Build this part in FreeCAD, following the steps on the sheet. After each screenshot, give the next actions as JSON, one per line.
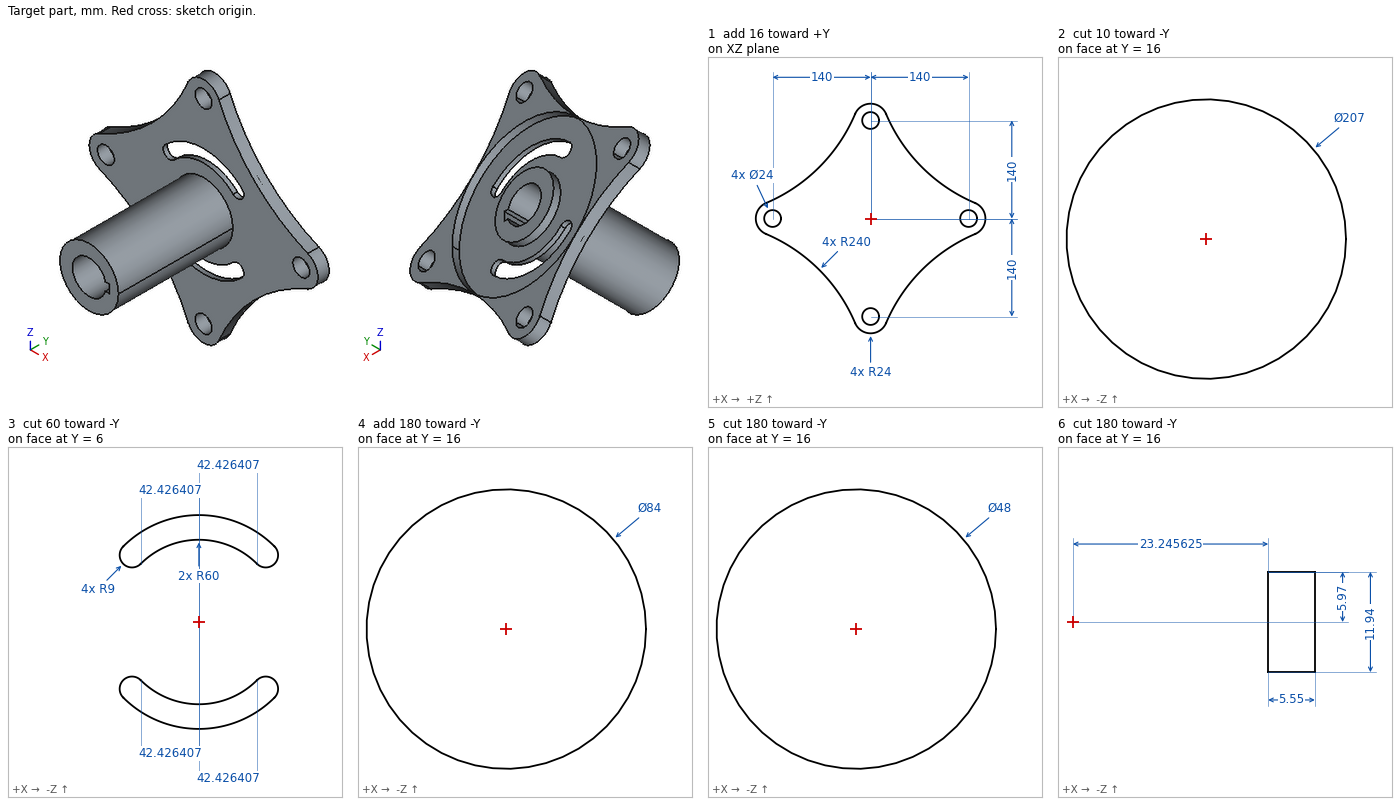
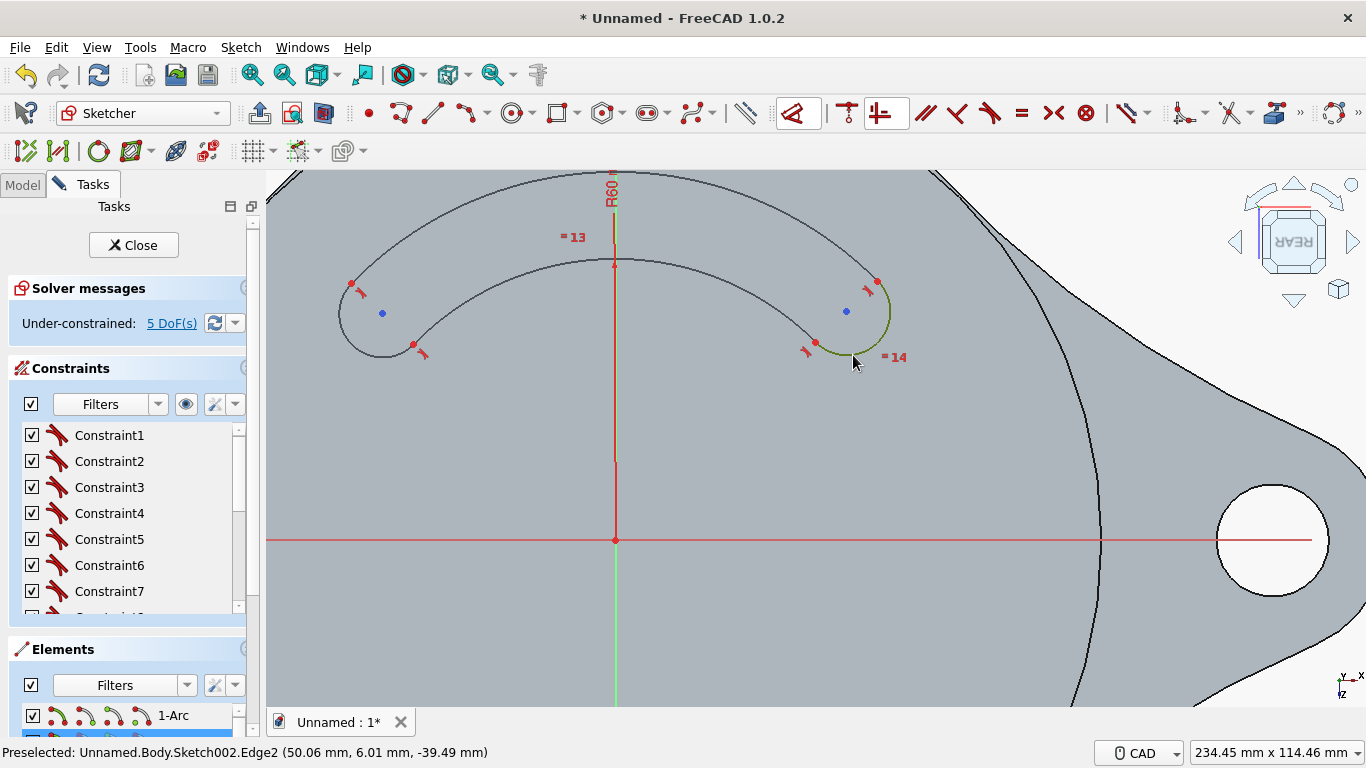
{"action": "key", "text": "k r"}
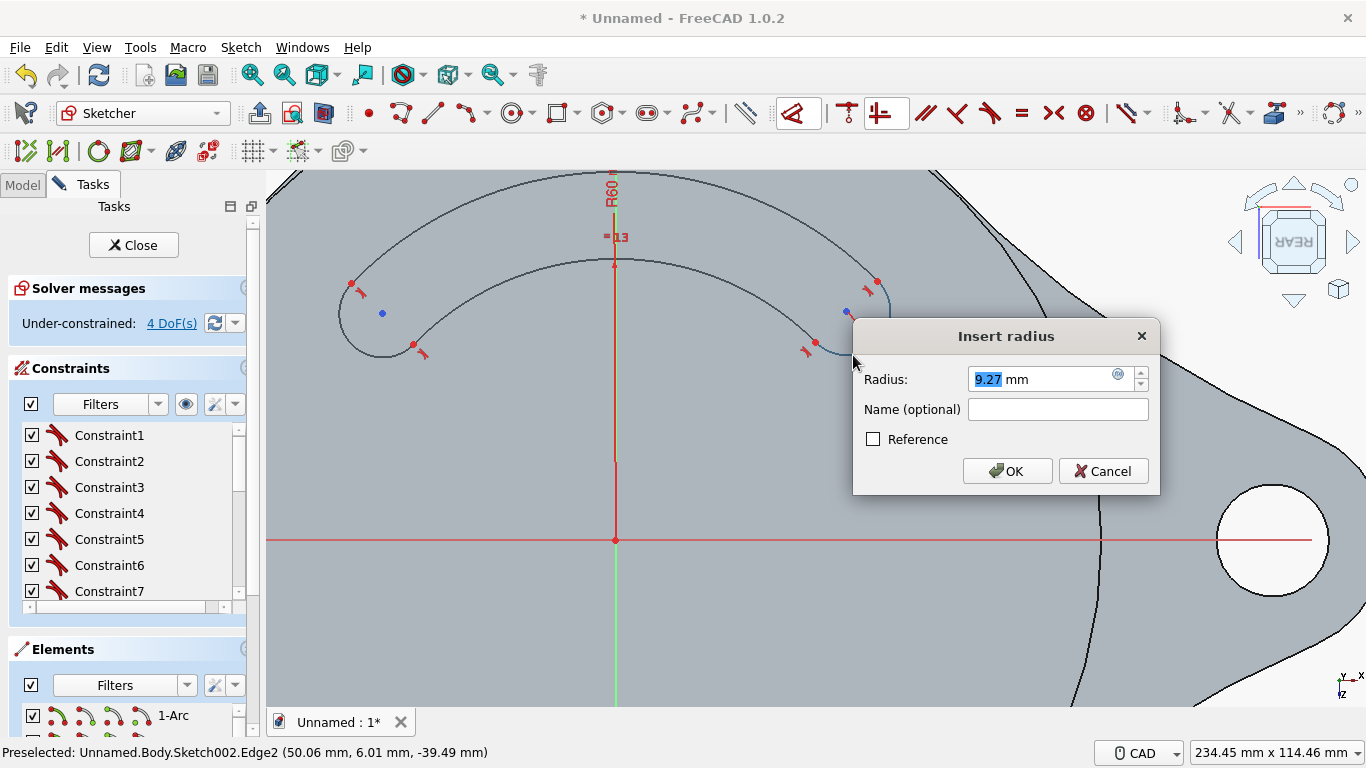
{"action": "type", "text": "9"}
{"action": "key", "text": "Return"}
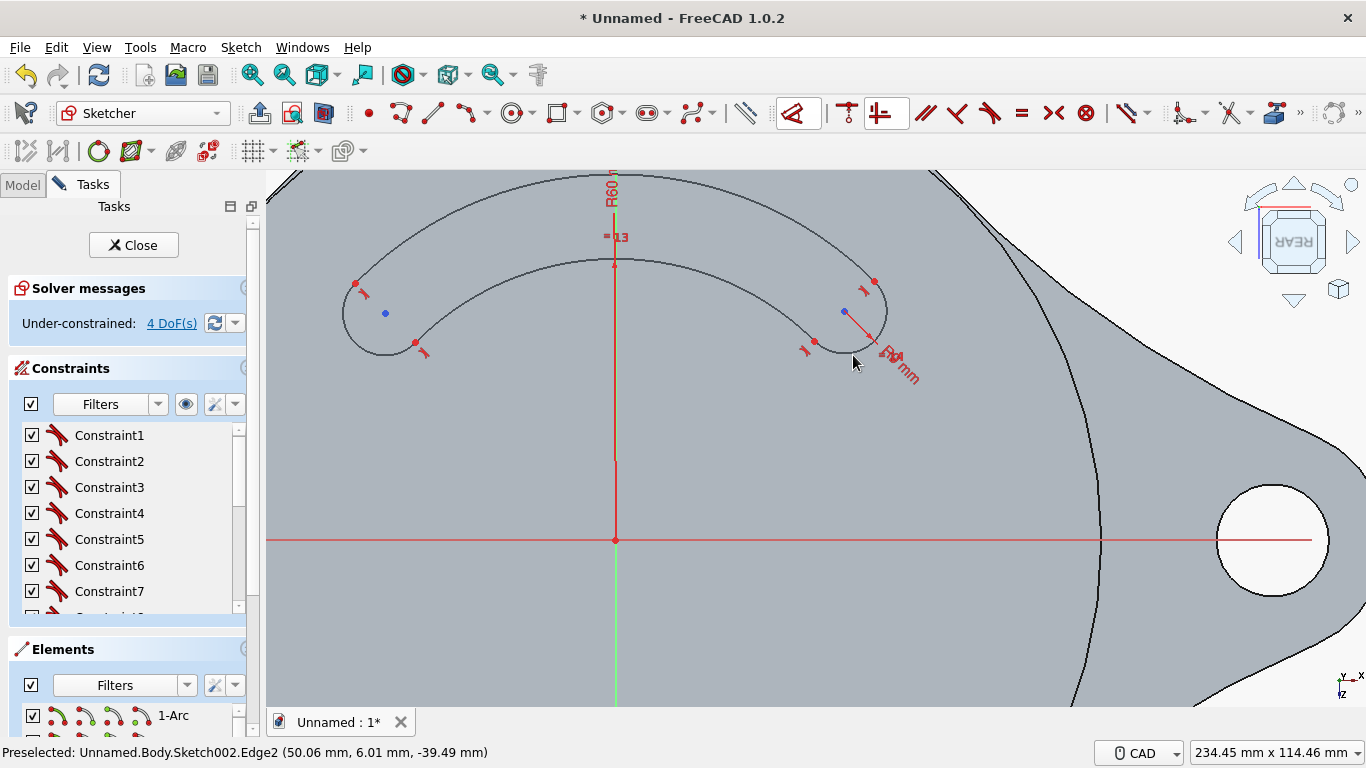
{"action": "left_click", "coordinate": [815, 341]}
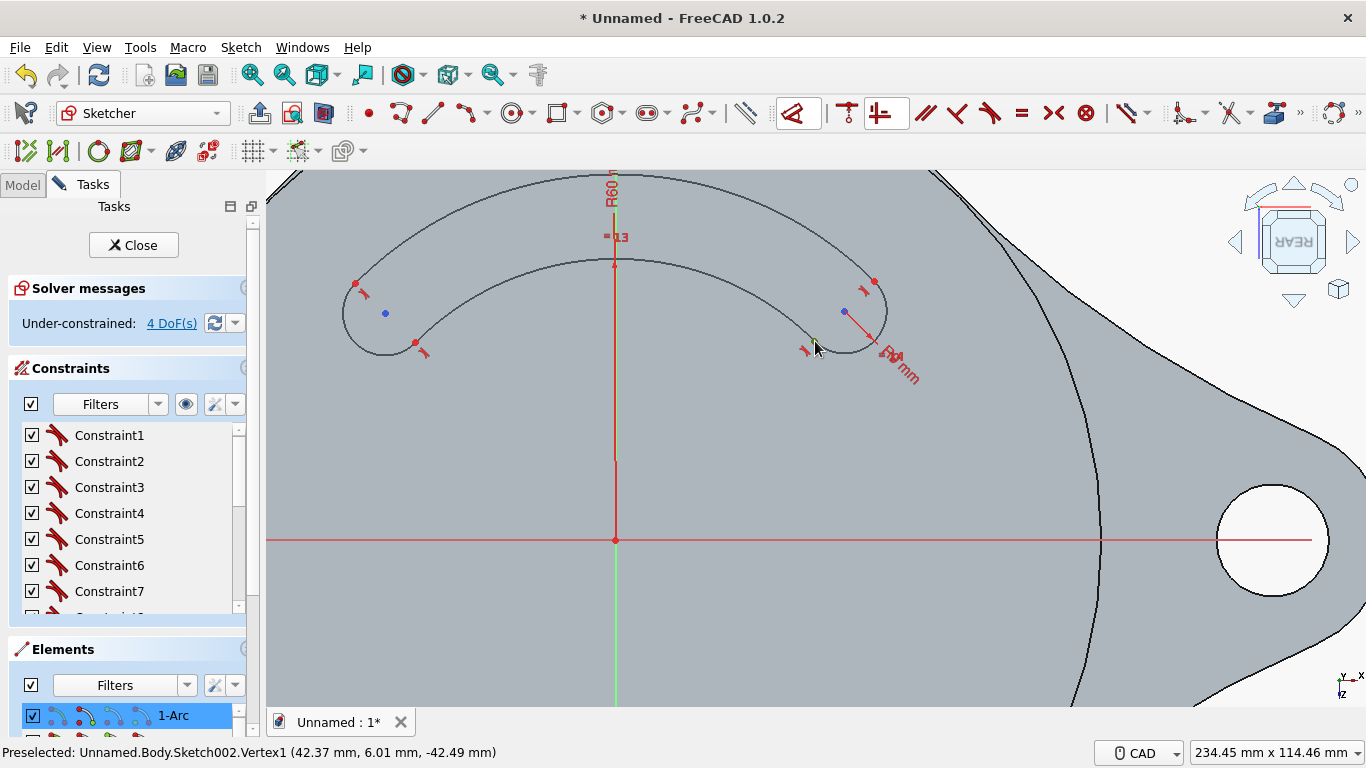
{"action": "left_click", "coordinate": [816, 114]}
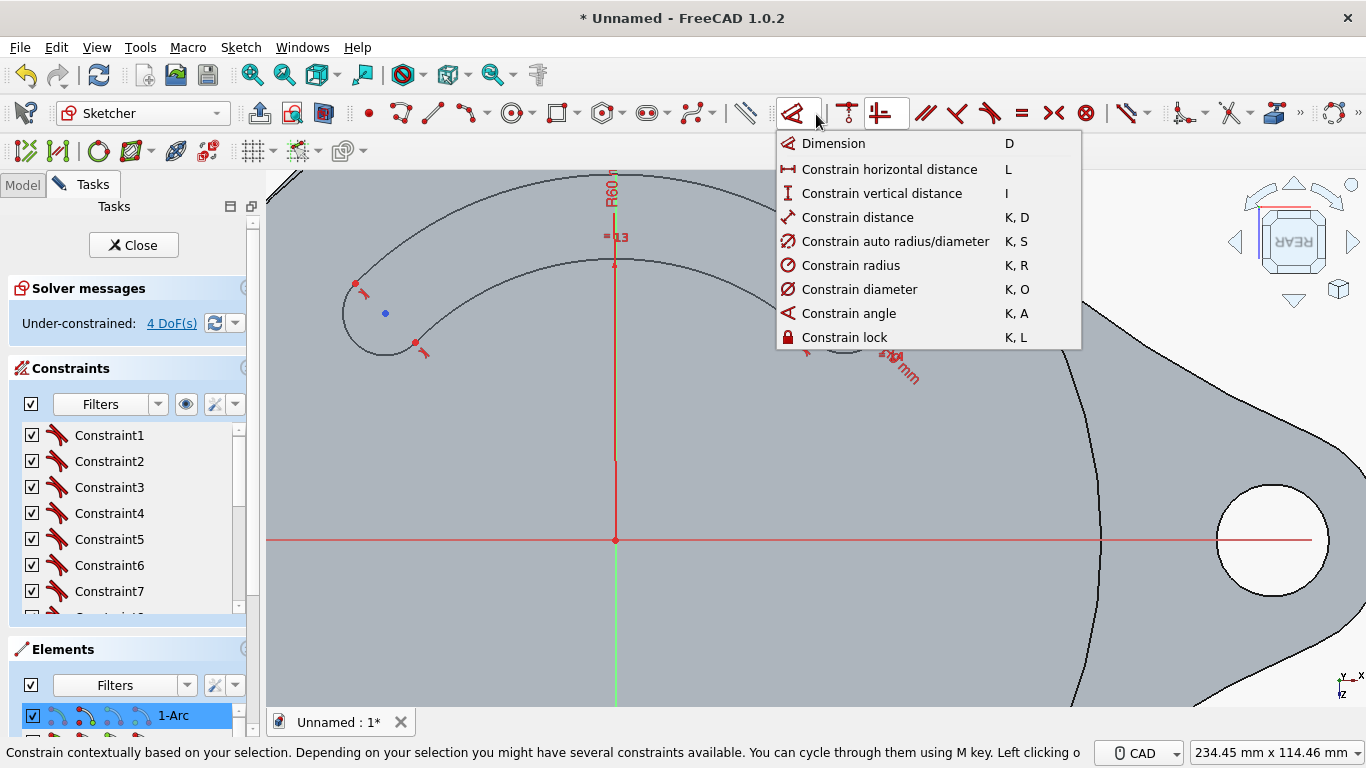
{"action": "left_click", "coordinate": [929, 169]}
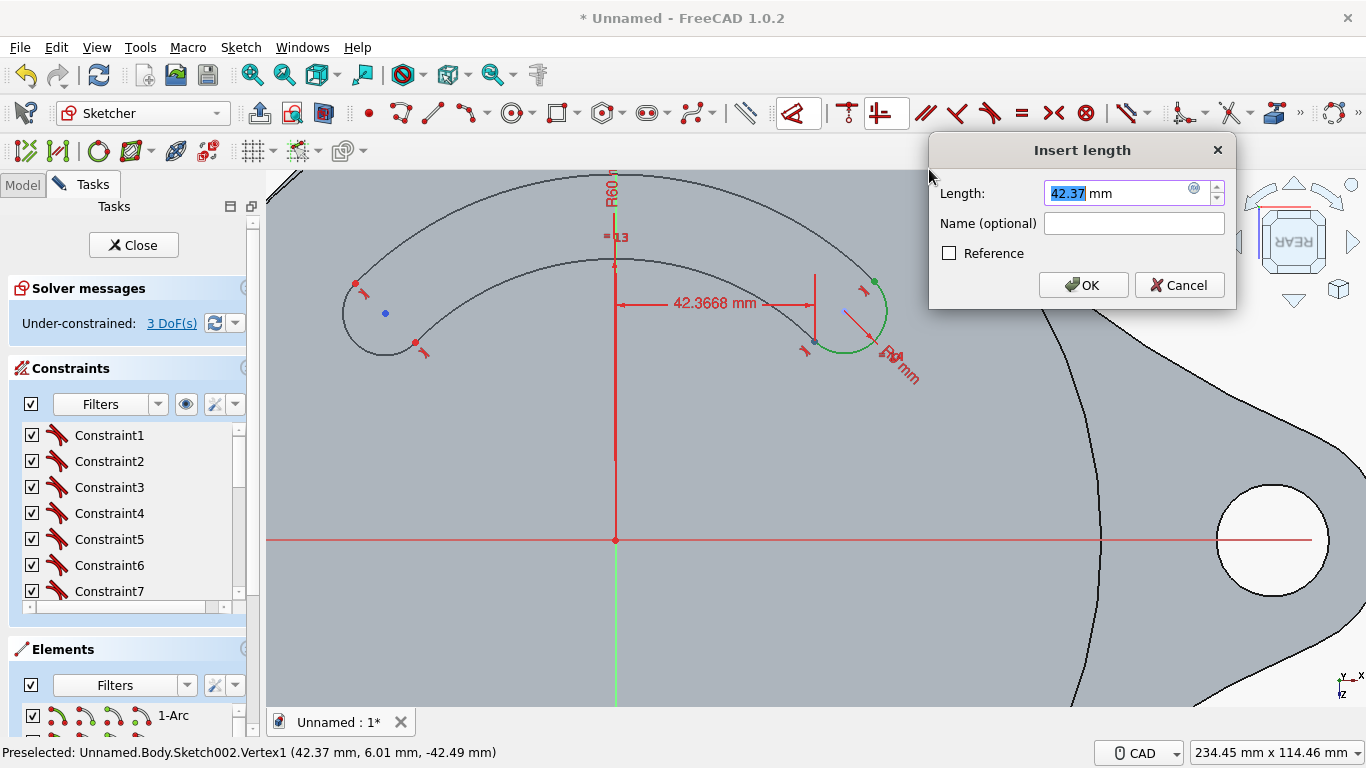
{"action": "type", "text": "42.426407"}
{"action": "key", "text": "Return"}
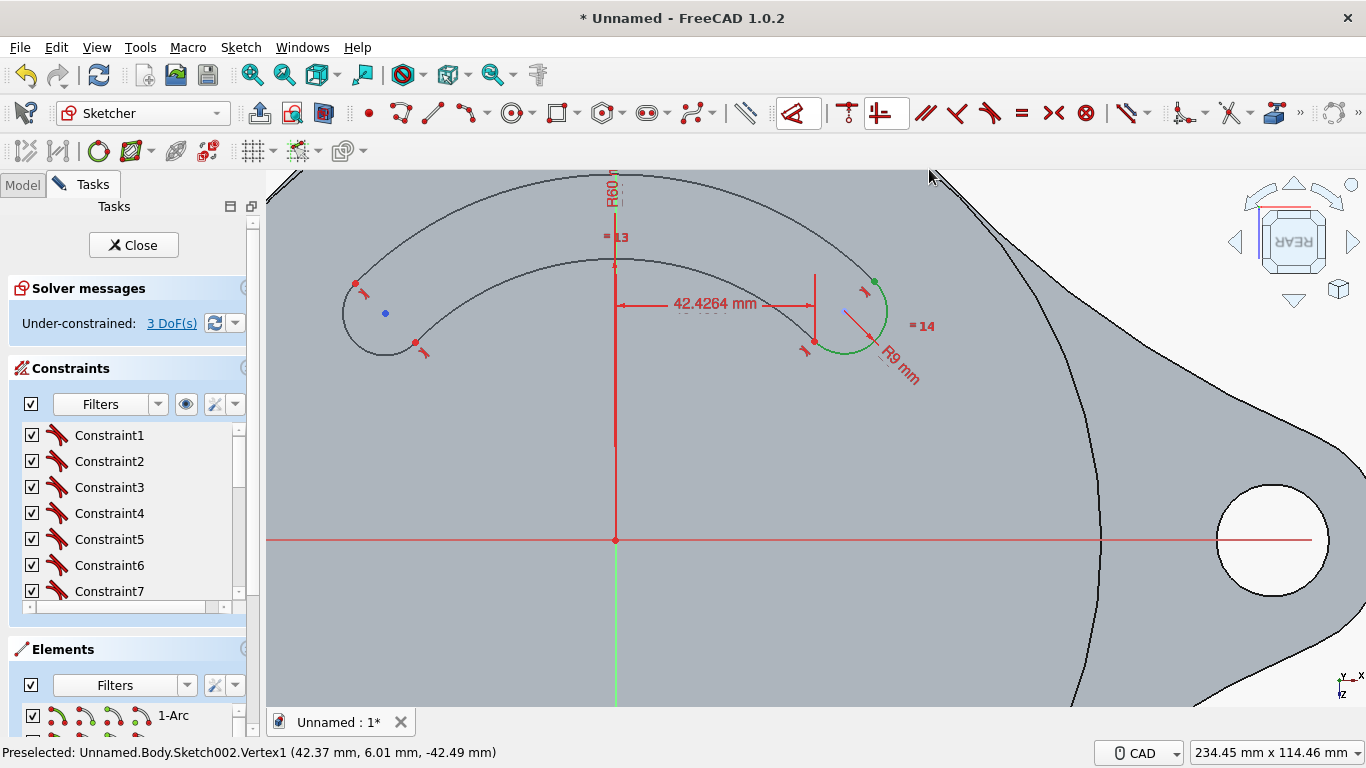
{"action": "left_click", "coordinate": [415, 343]}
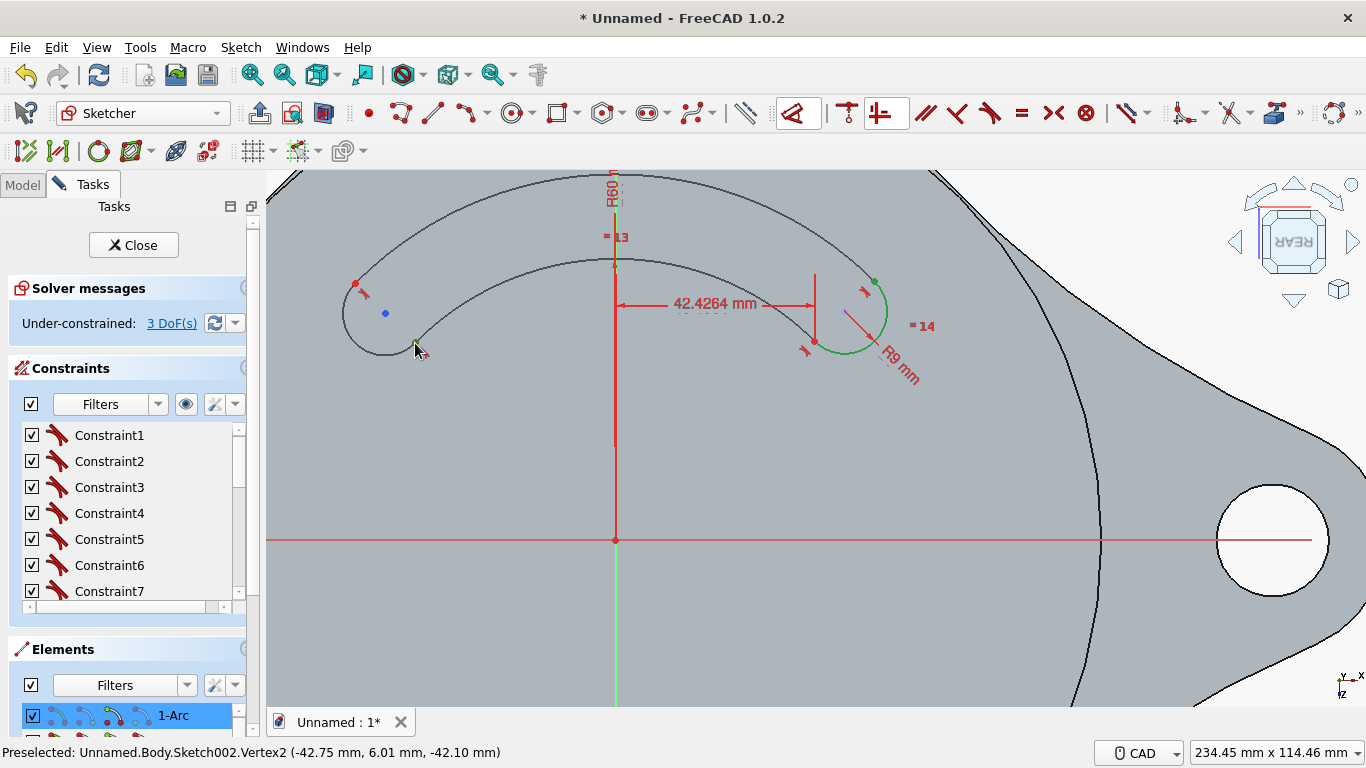
{"action": "left_click", "coordinate": [816, 114]}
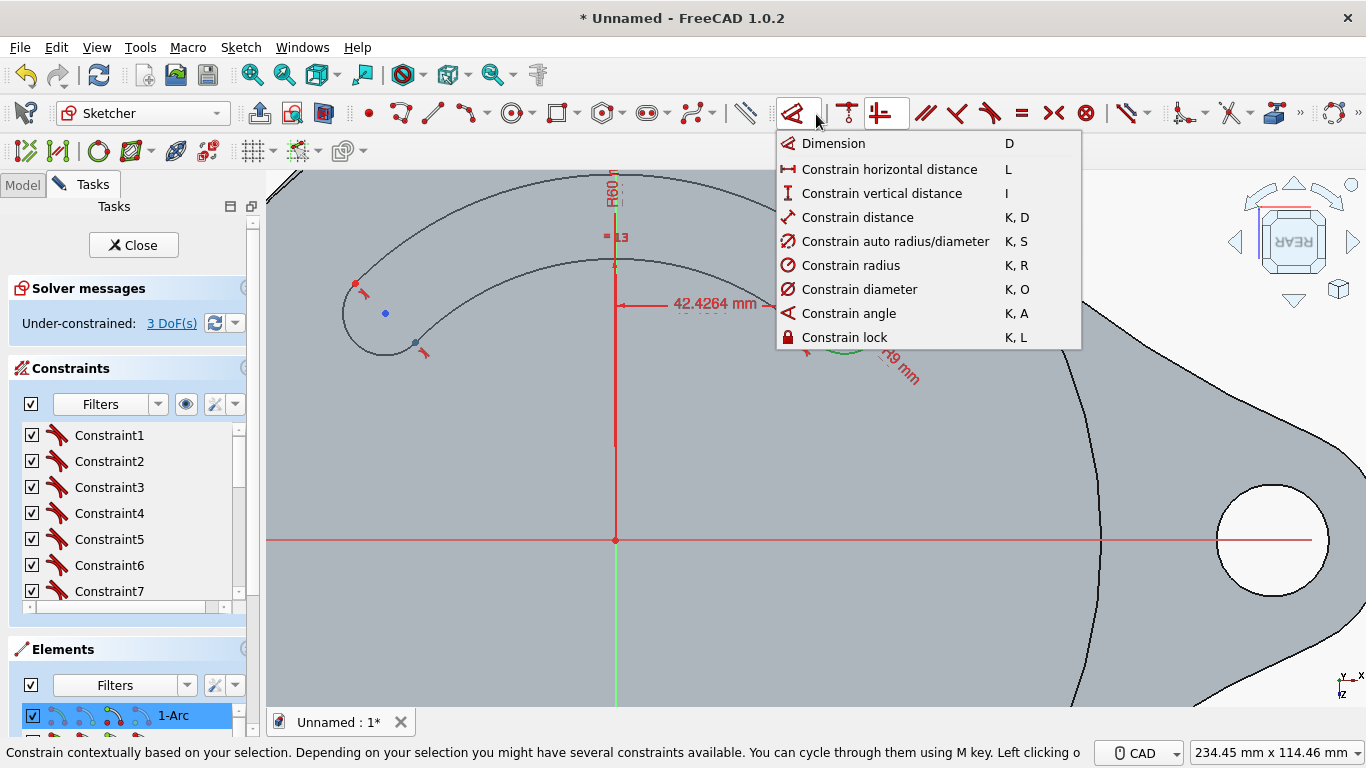
{"action": "left_click", "coordinate": [929, 169]}